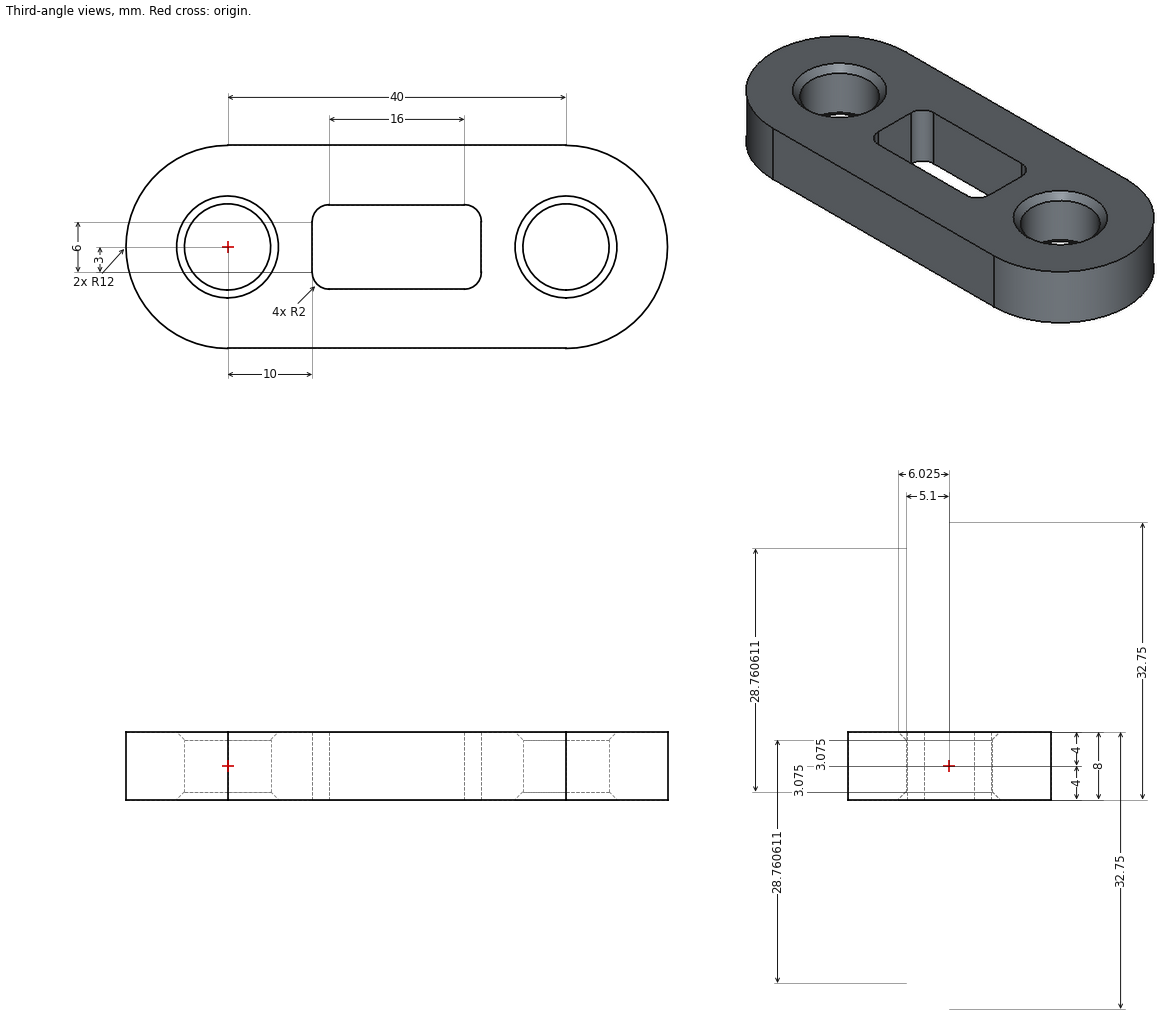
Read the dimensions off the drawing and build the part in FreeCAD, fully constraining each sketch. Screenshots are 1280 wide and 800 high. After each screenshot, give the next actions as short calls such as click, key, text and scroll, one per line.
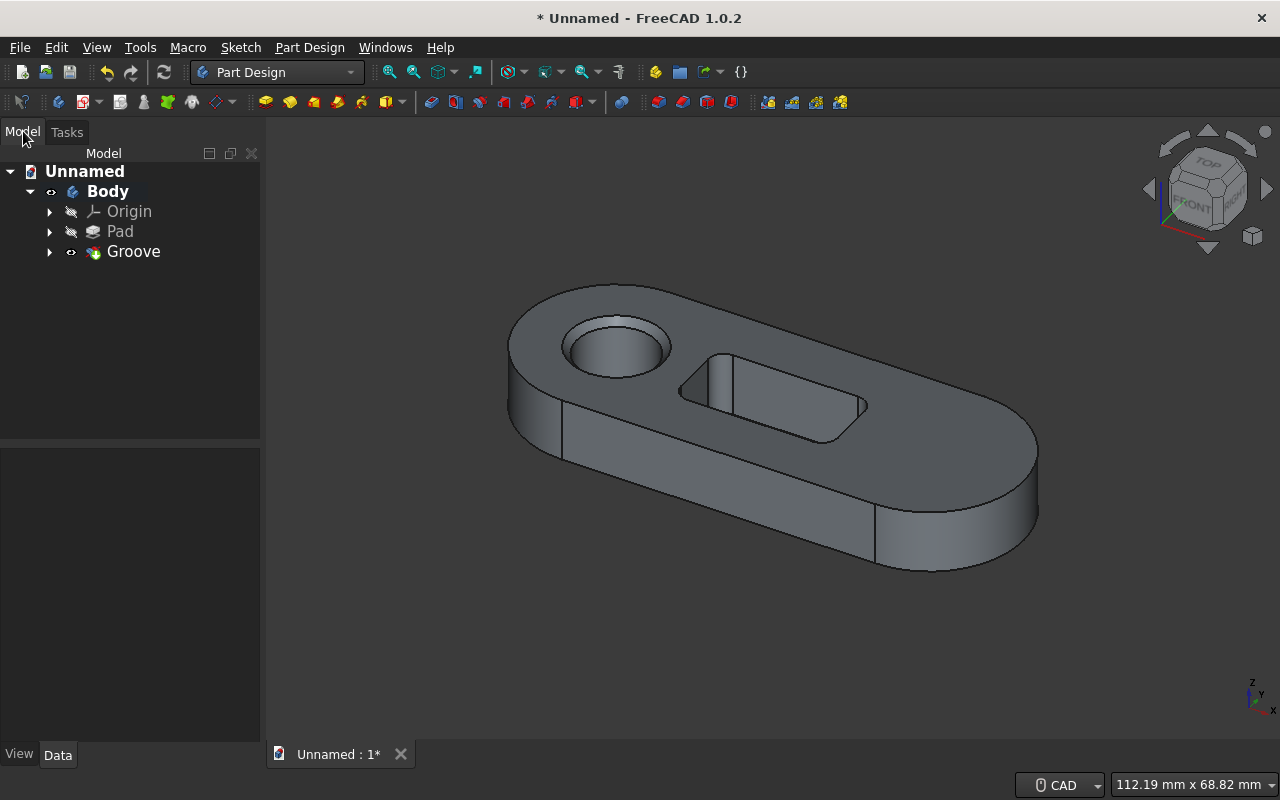
click(116, 252)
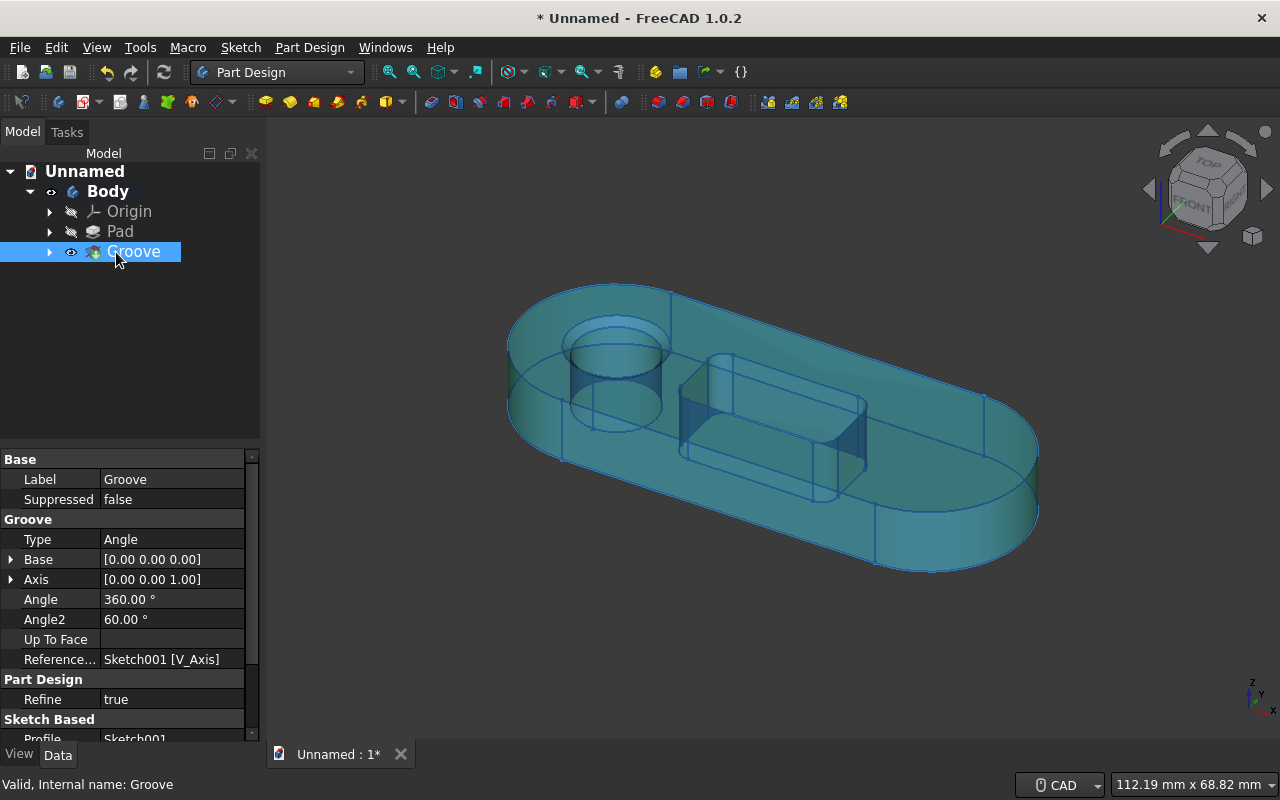
click(768, 102)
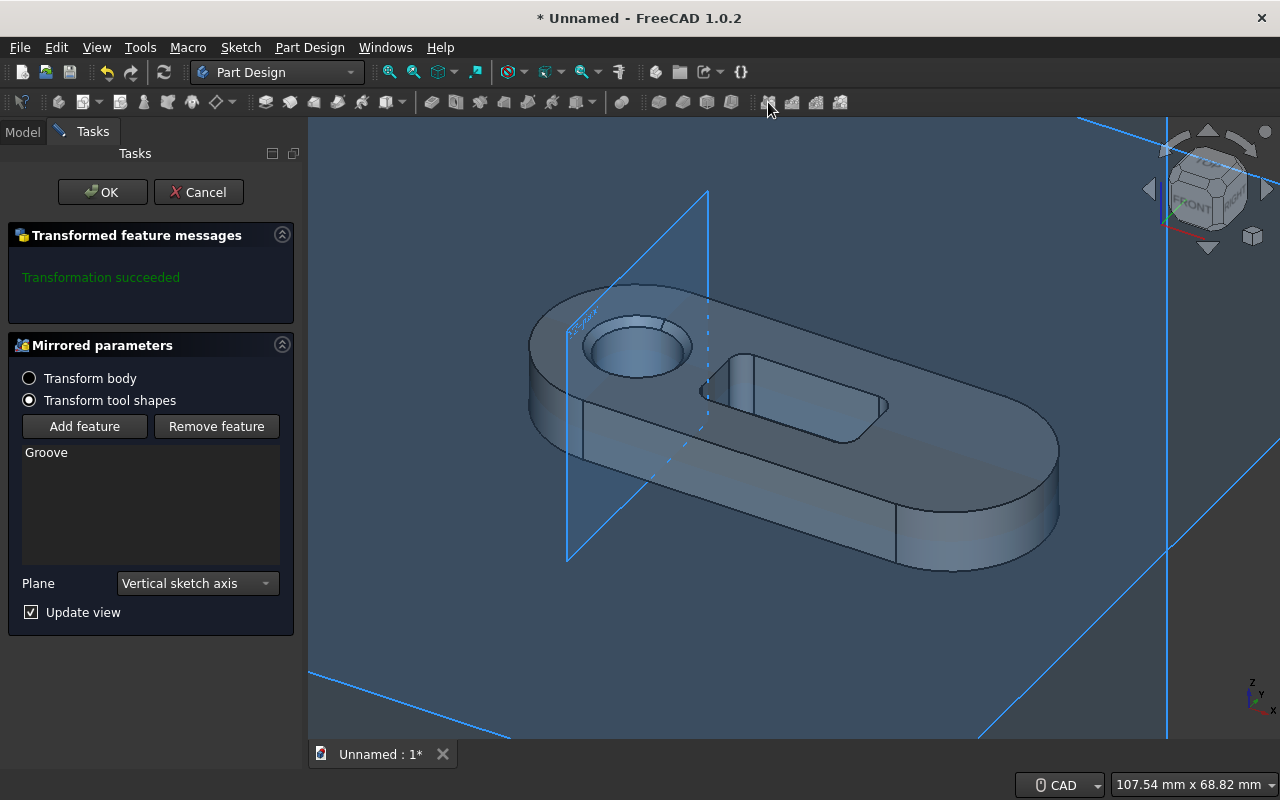
click(198, 584)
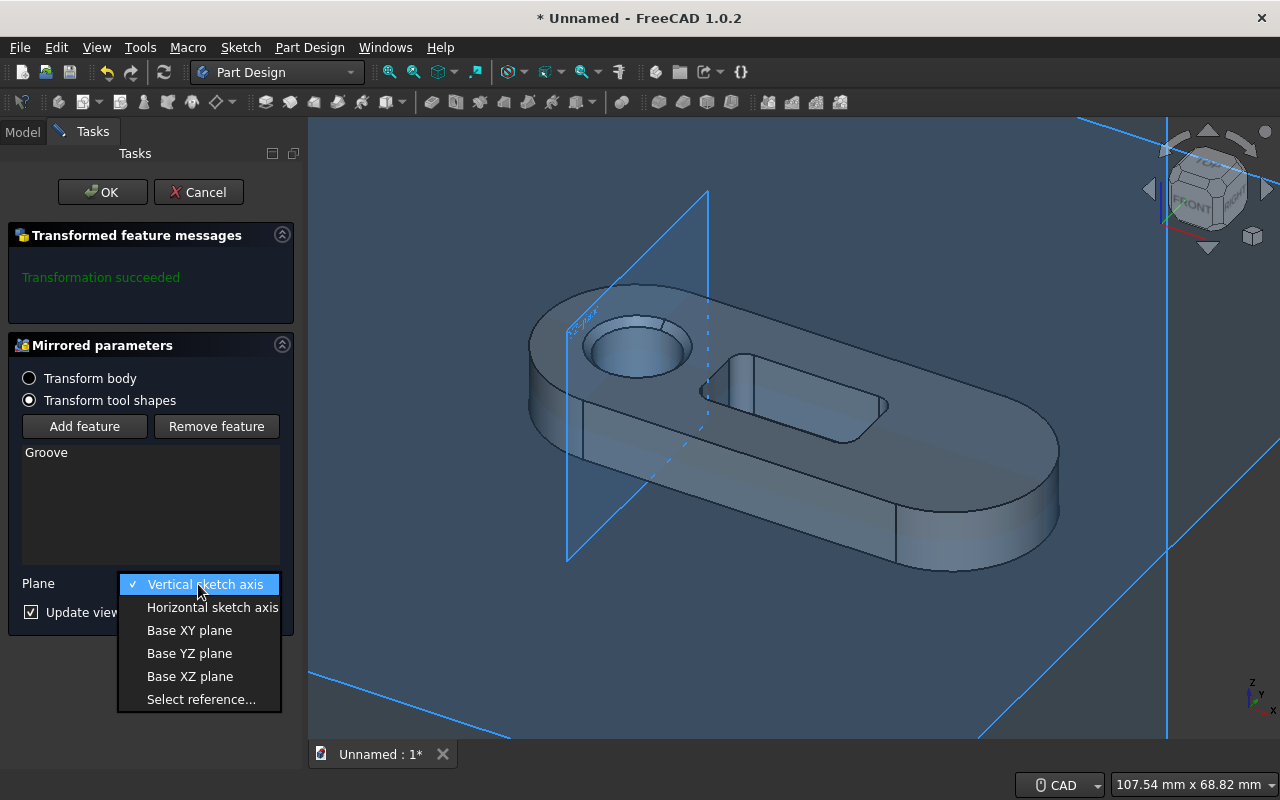
click(198, 630)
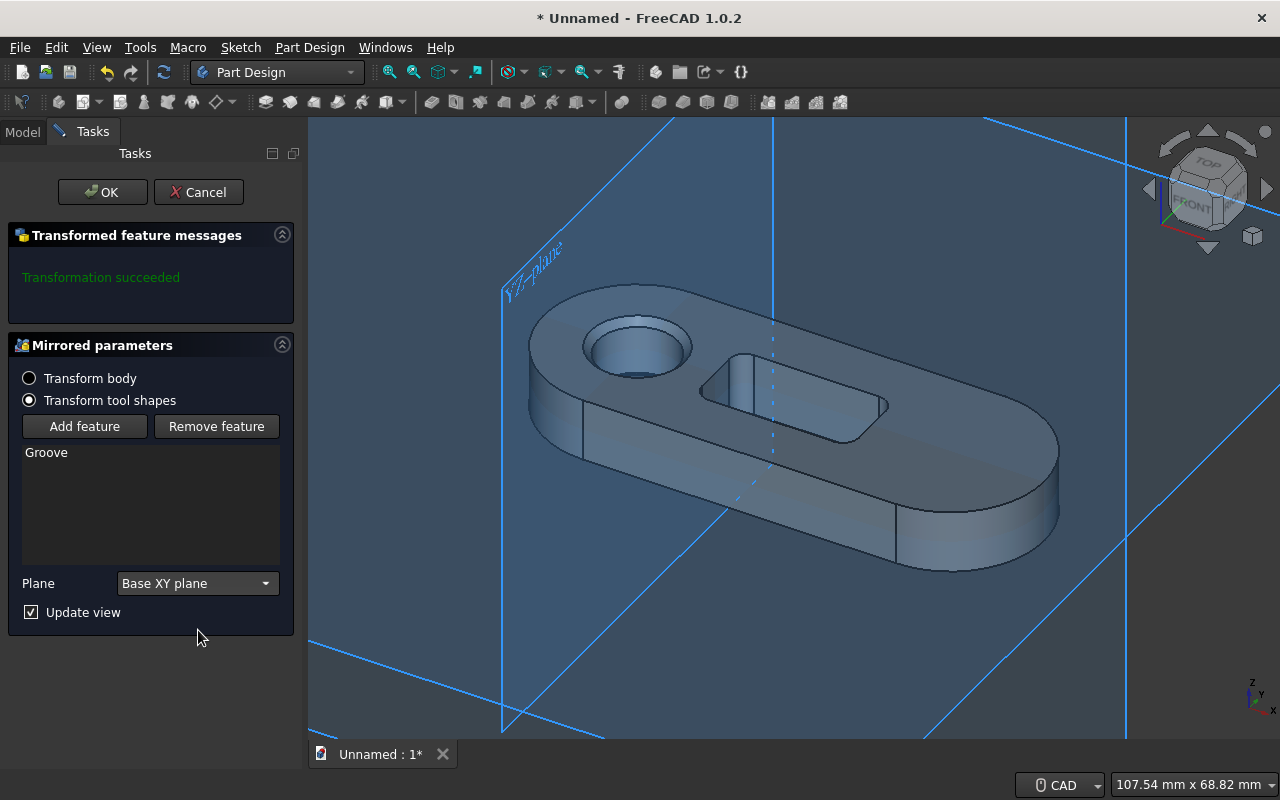
click(103, 192)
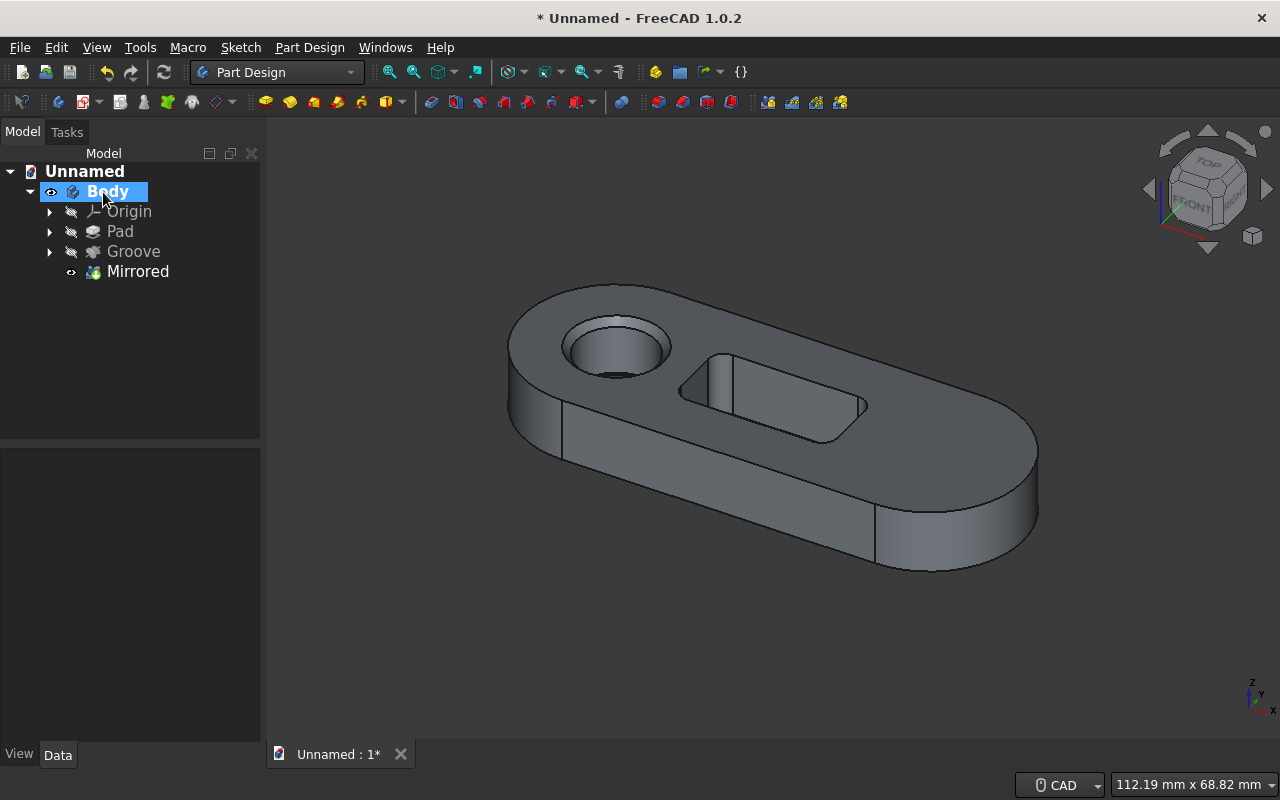
click(50, 212)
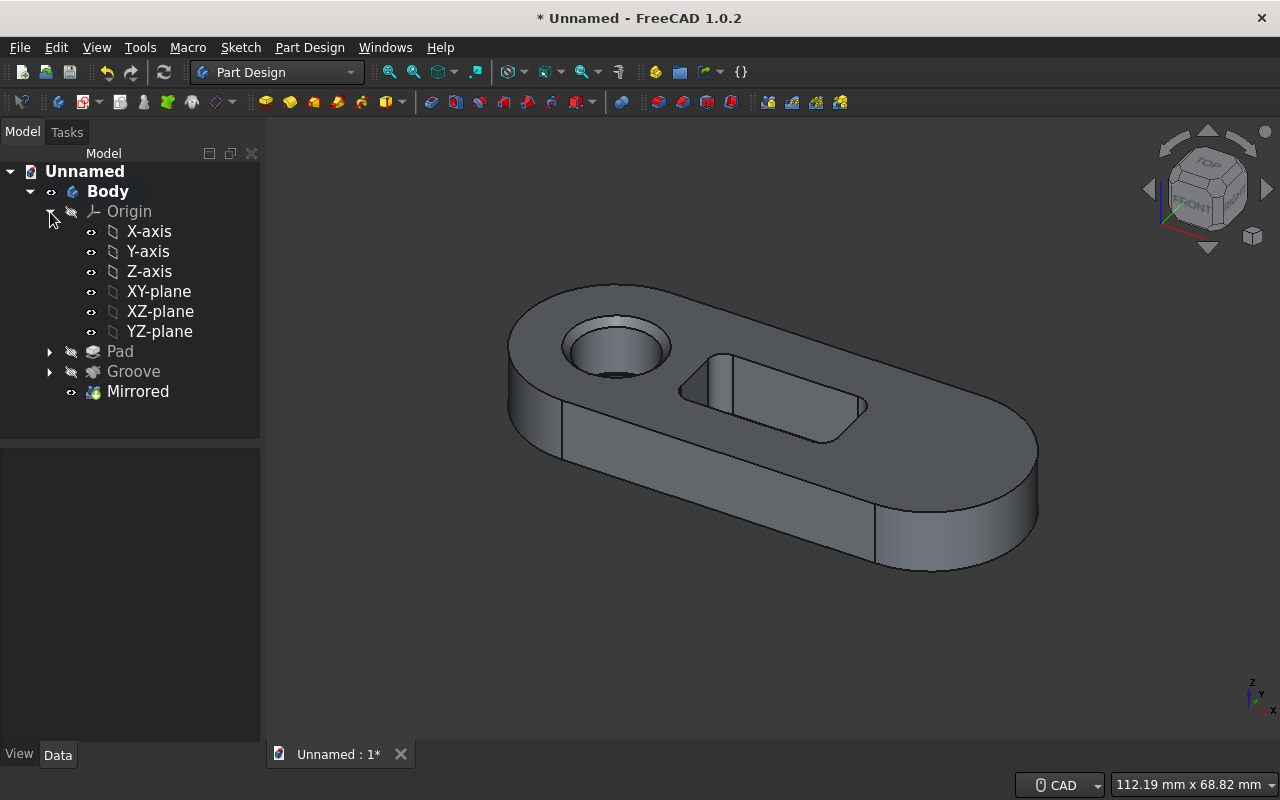
click(136, 332)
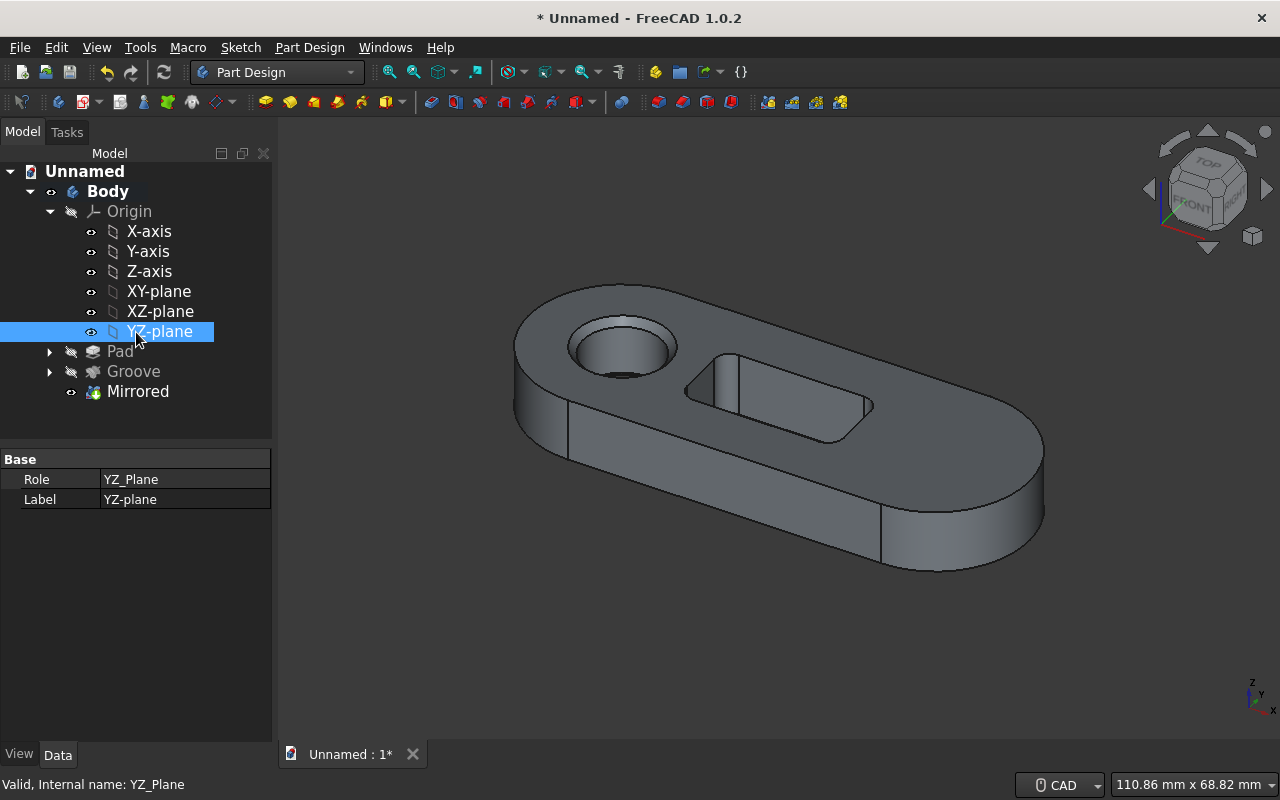
click(216, 102)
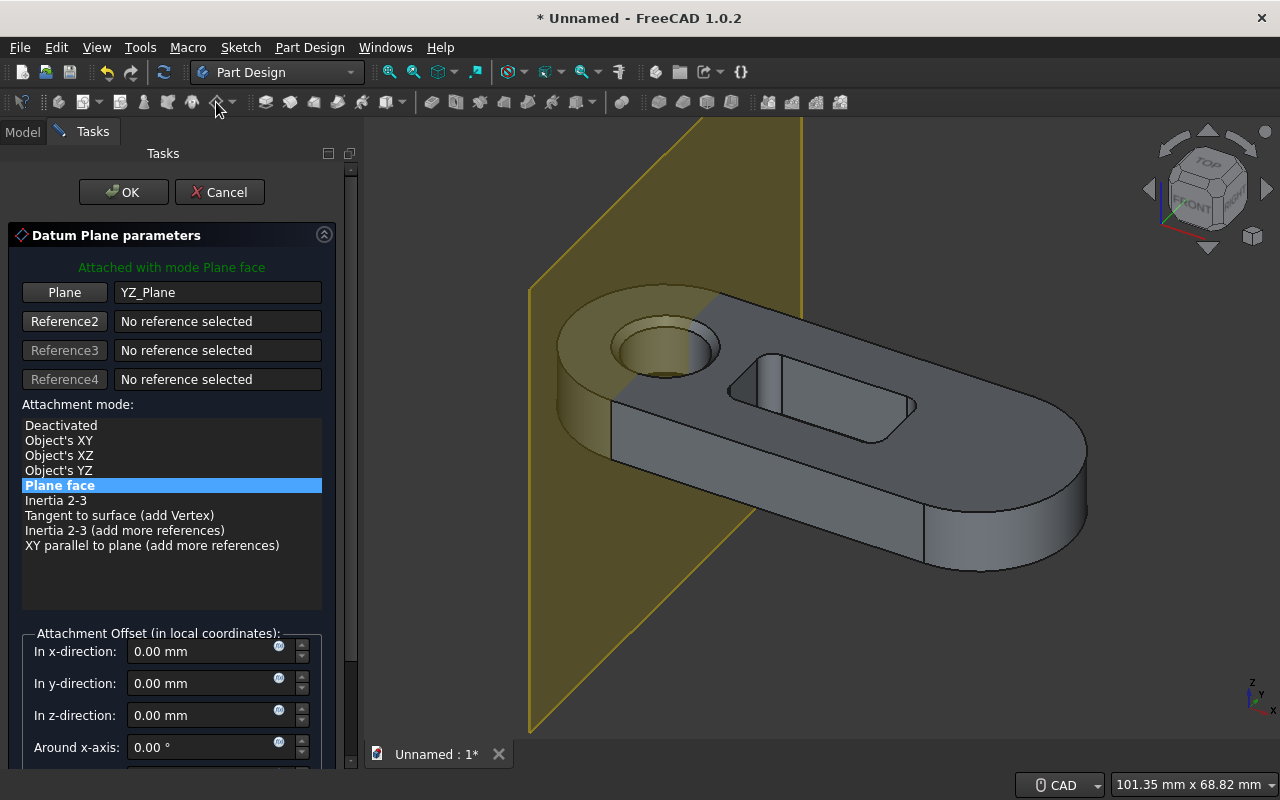
triple_click(210, 715)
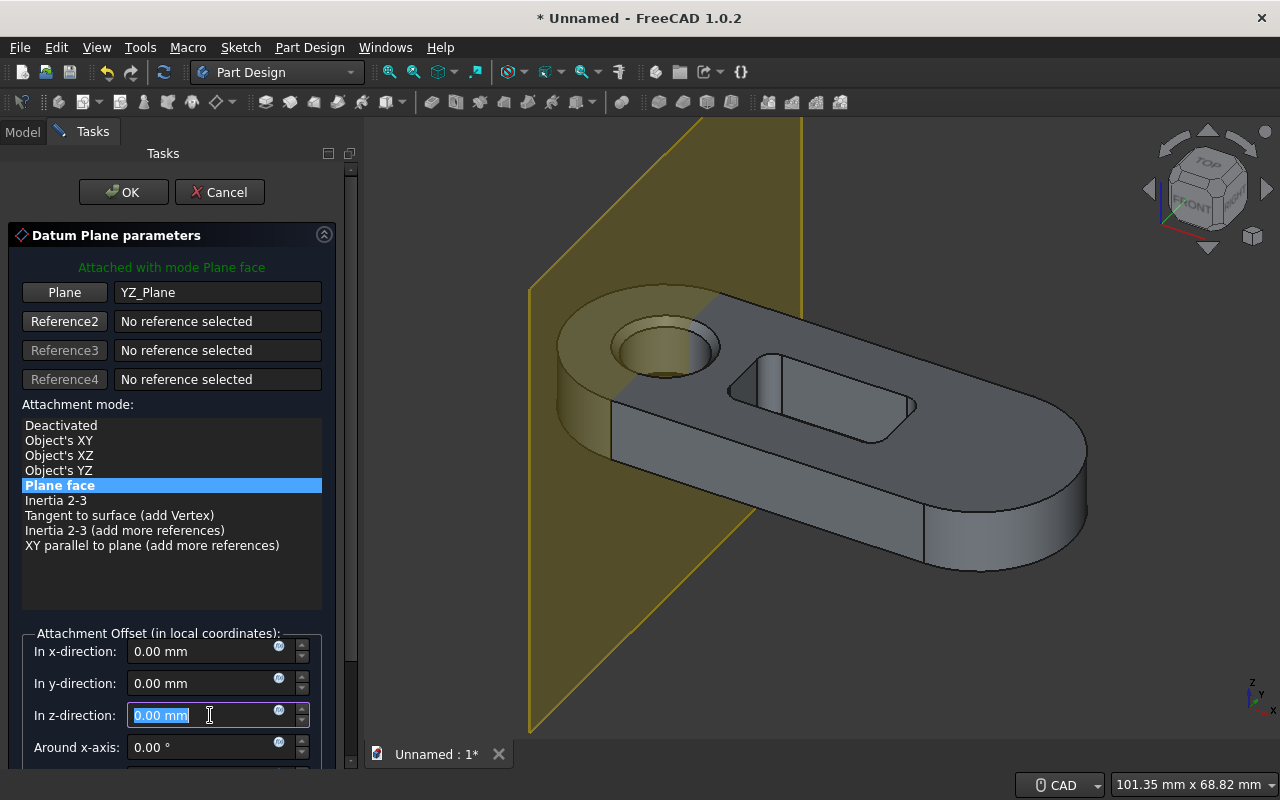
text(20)
key(Tab)